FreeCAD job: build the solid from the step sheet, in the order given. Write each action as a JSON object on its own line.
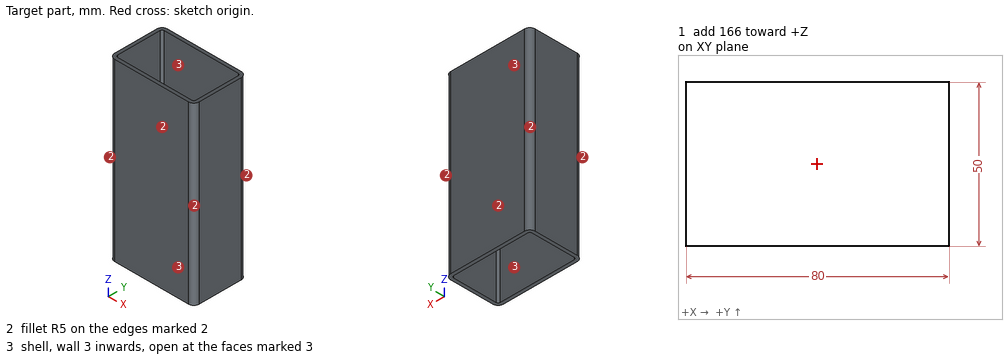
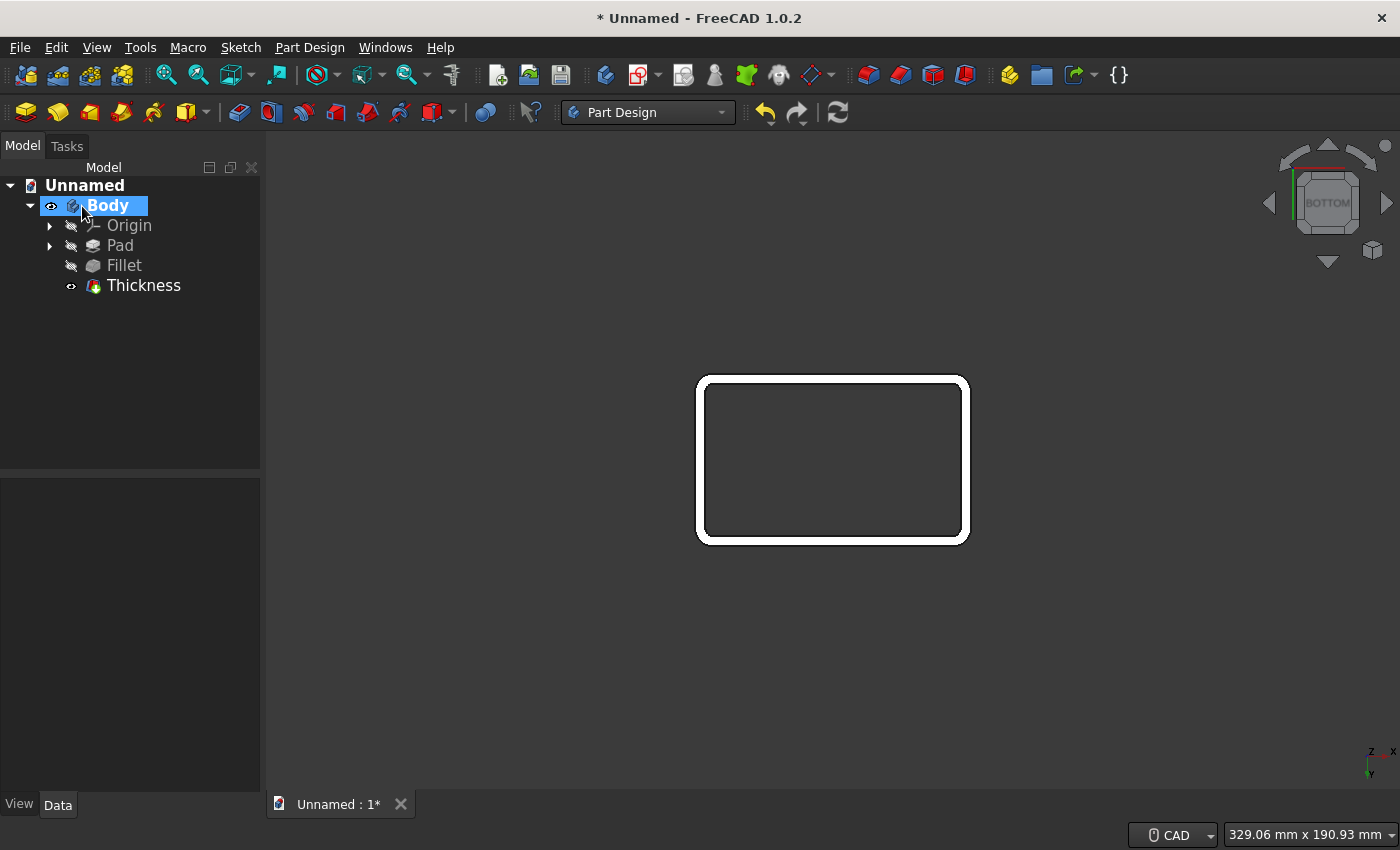
{"action": "key", "text": "0"}